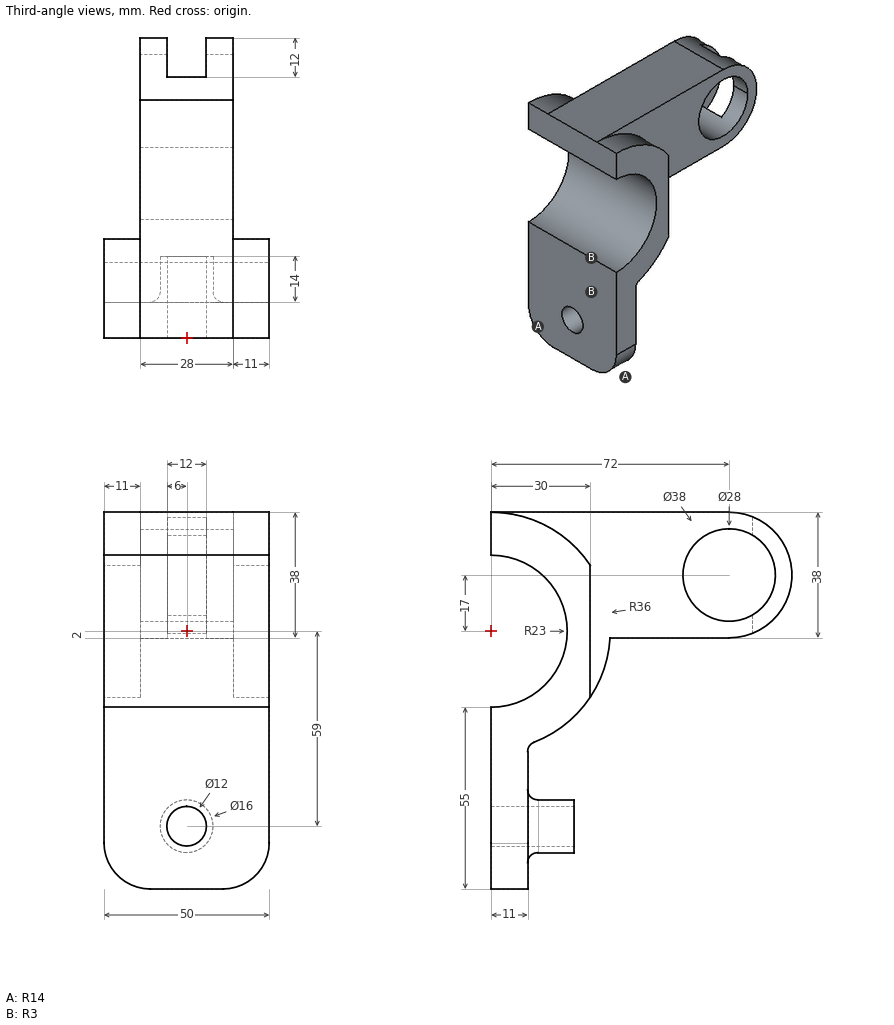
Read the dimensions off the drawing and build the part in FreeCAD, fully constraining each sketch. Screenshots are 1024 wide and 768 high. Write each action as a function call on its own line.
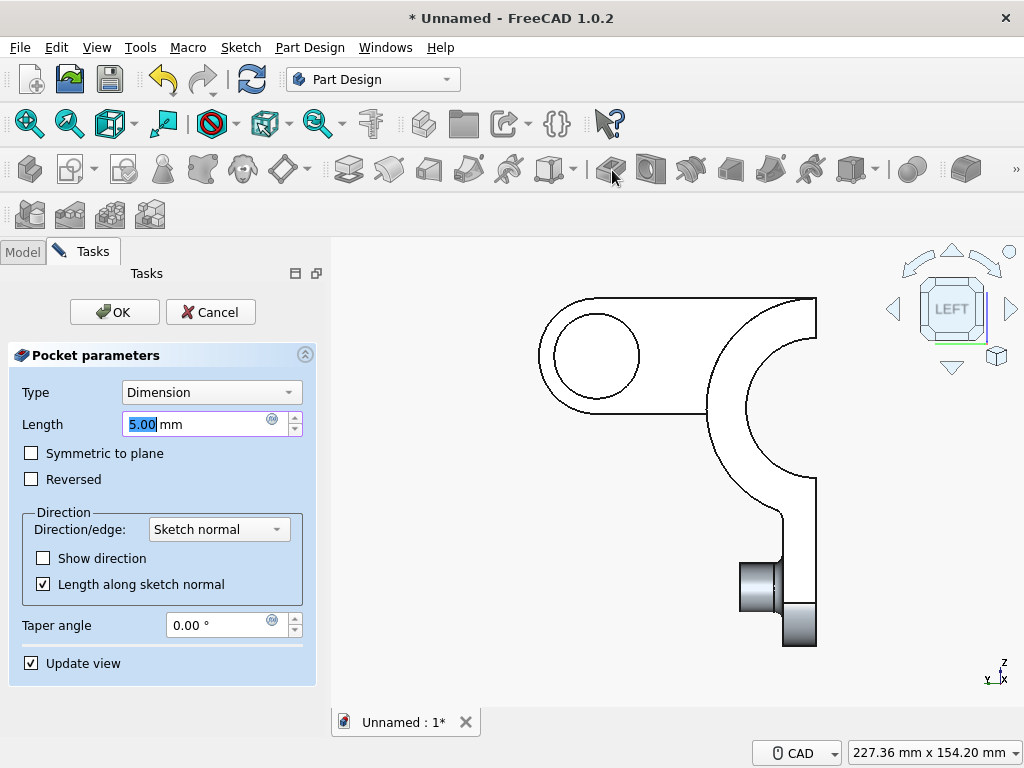
click(212, 392)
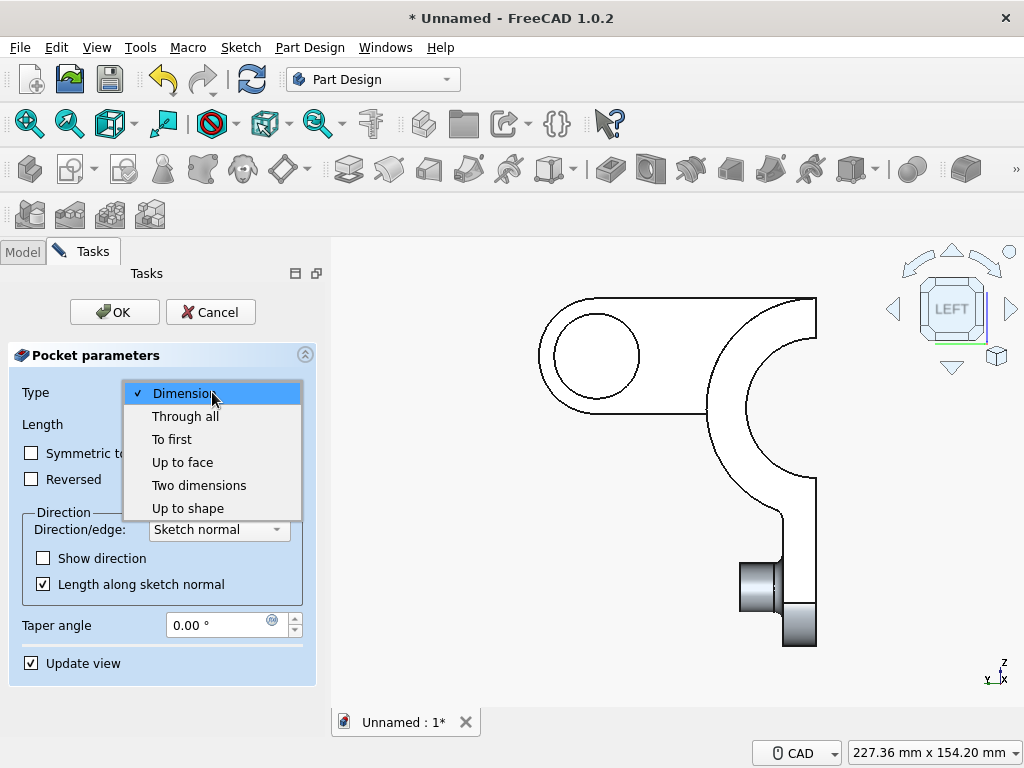
click(212, 416)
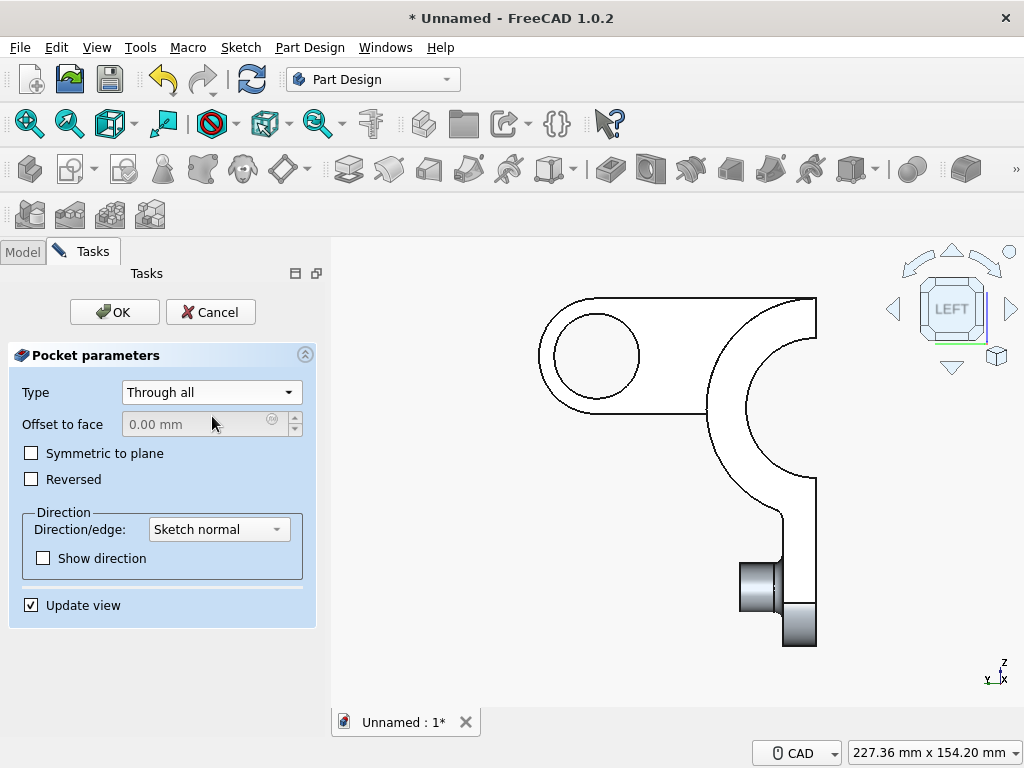
click(115, 312)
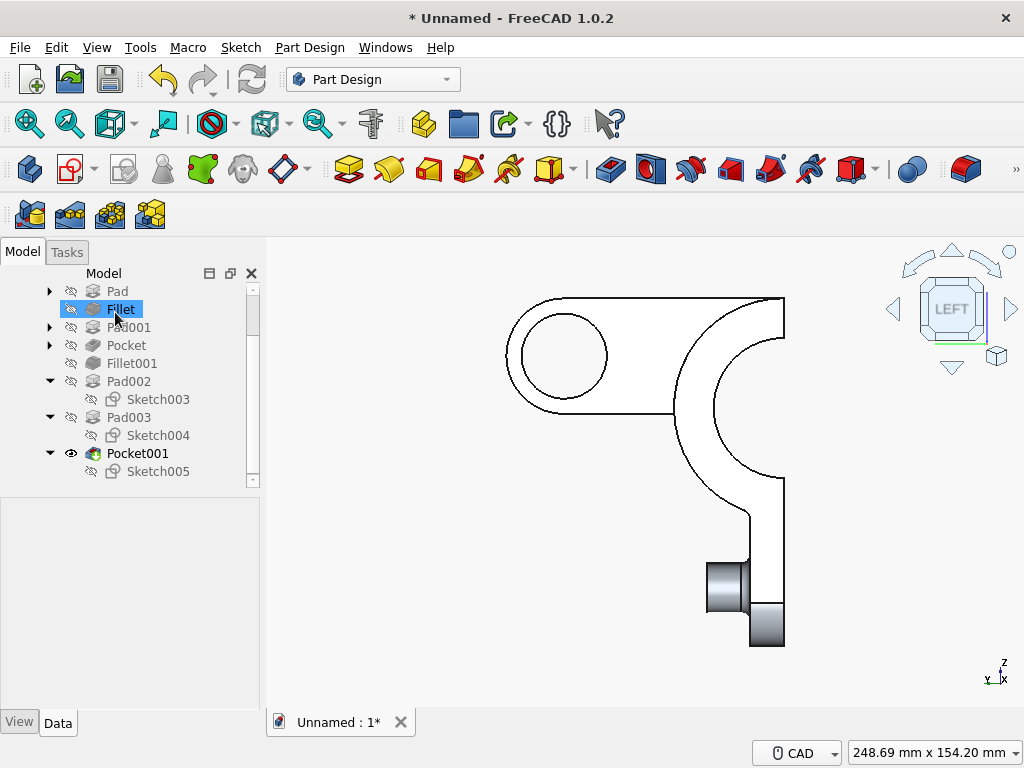
click(645, 339)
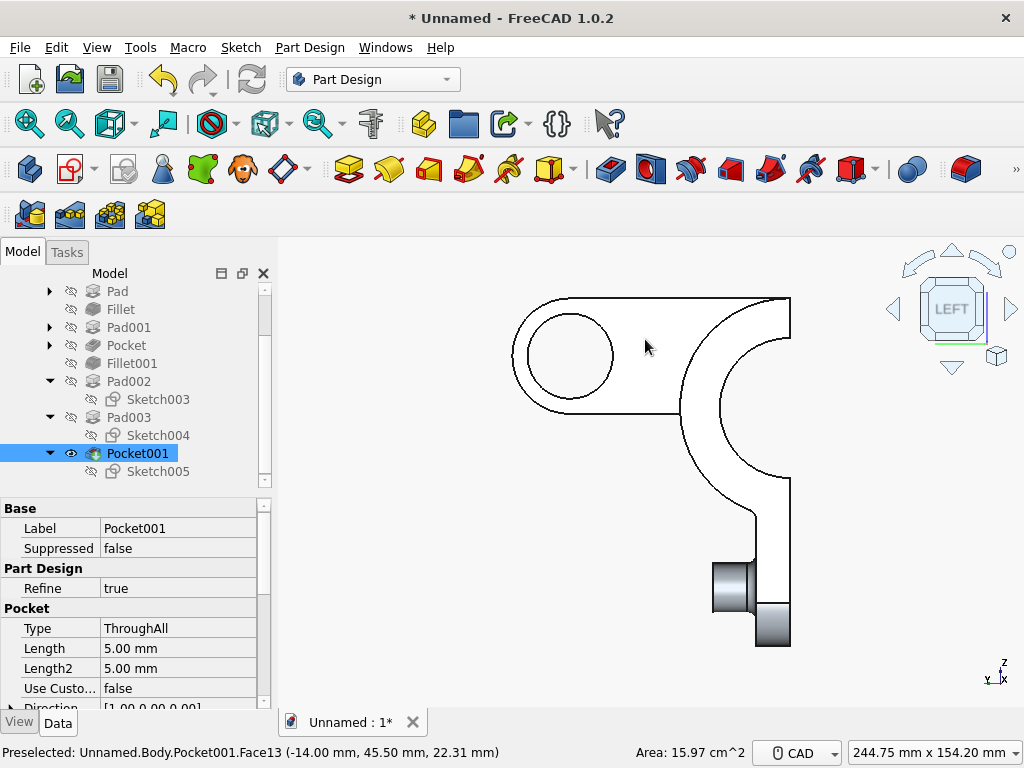
click(70, 170)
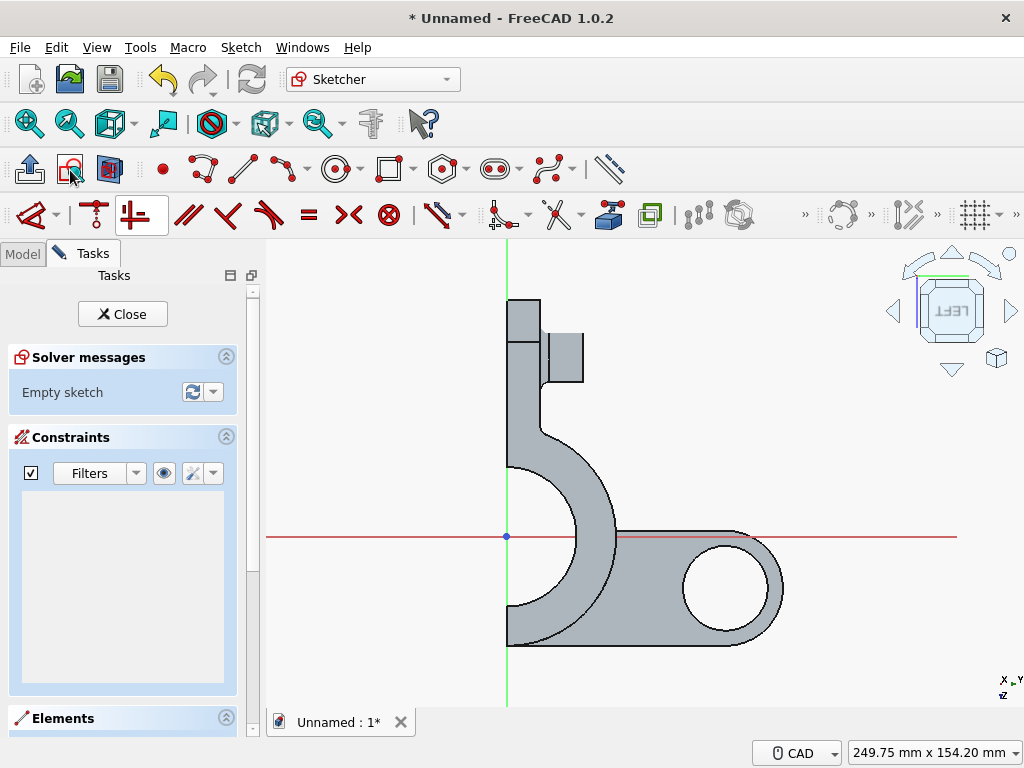
scroll(549, 589, up, 4)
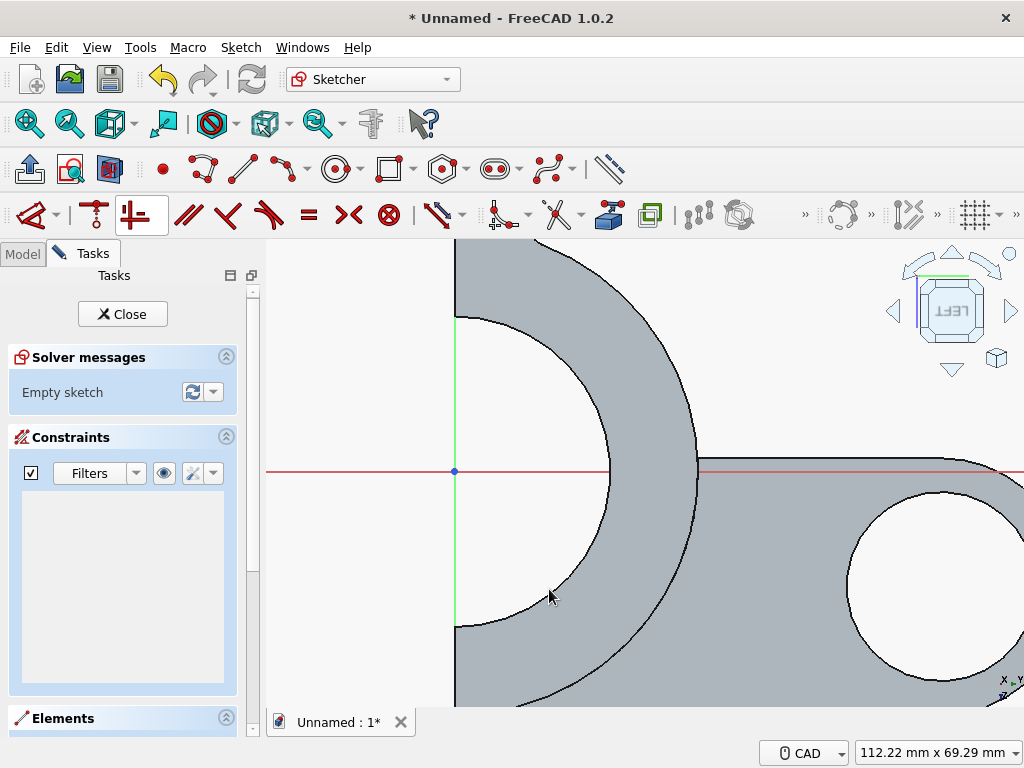
click(244, 170)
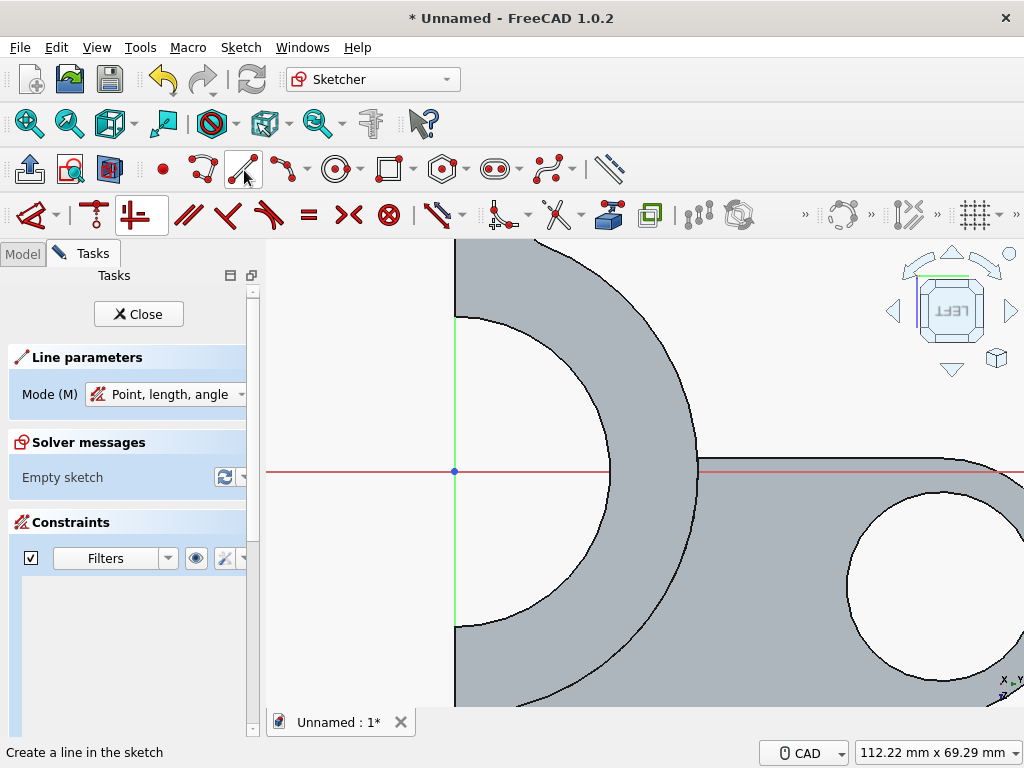
click(657, 337)
click(657, 606)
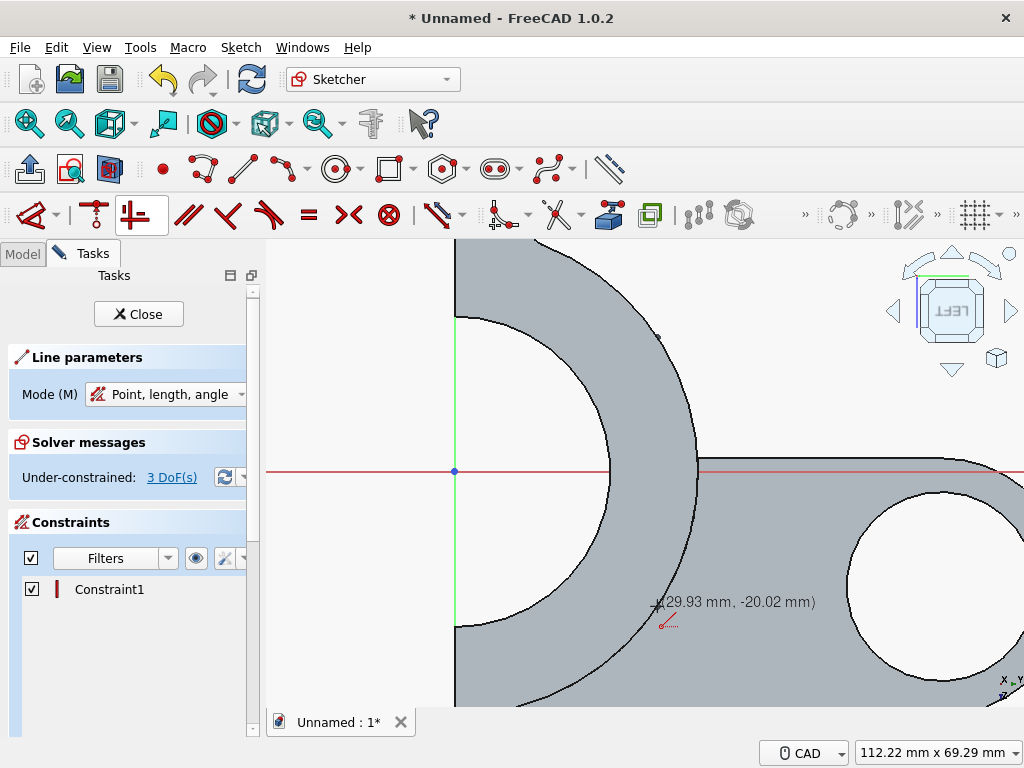
click(284, 170)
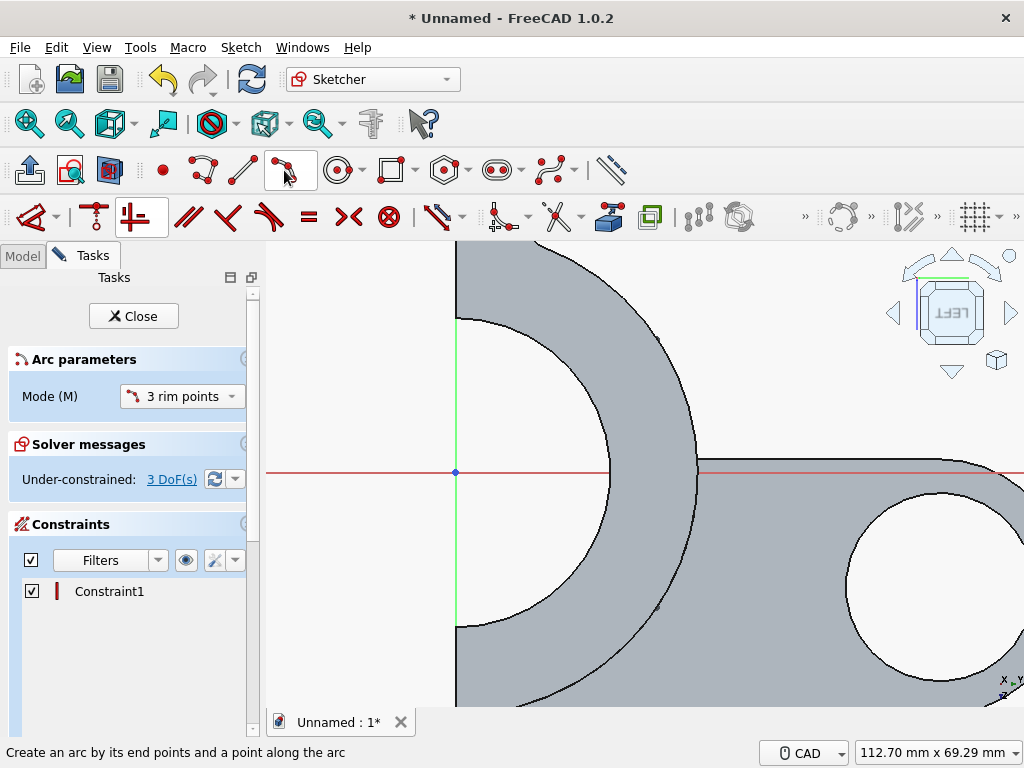
click(657, 607)
click(657, 340)
click(696, 501)
key(Escape)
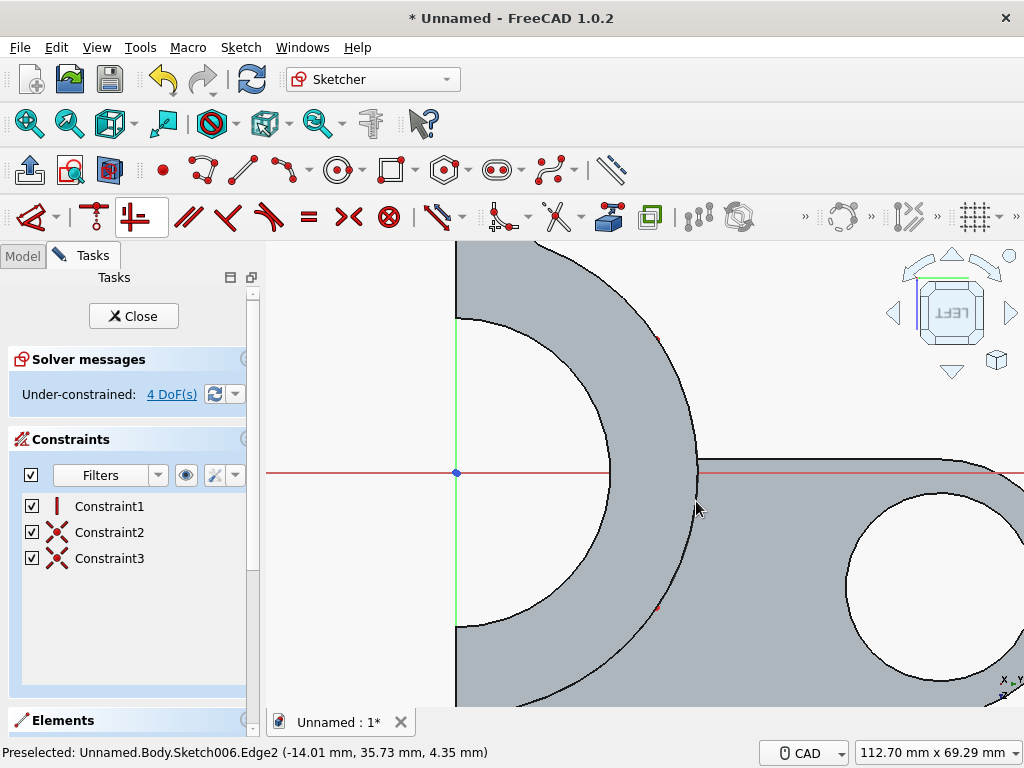
drag(446, 463, 467, 484)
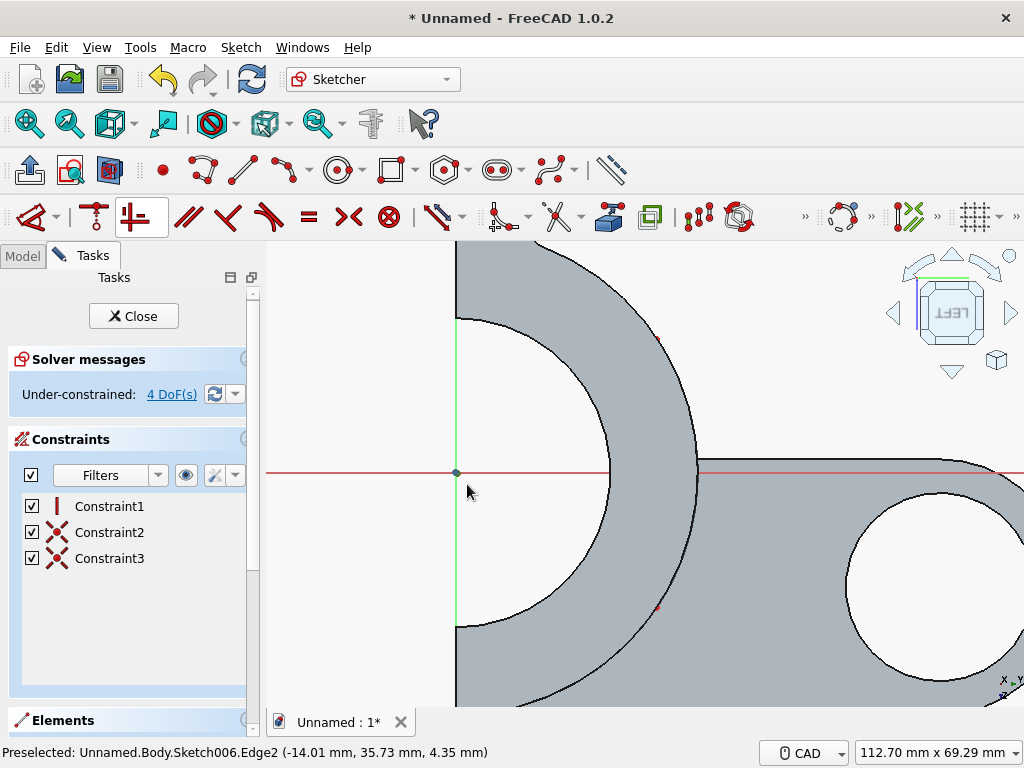
click(94, 218)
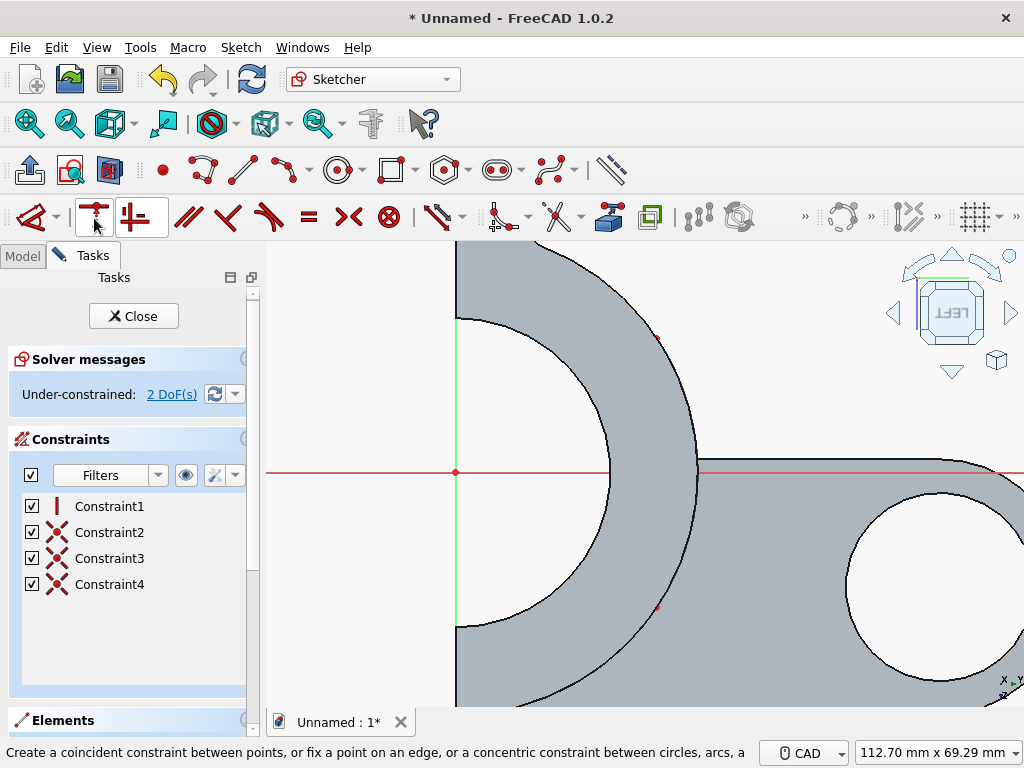
click(32, 218)